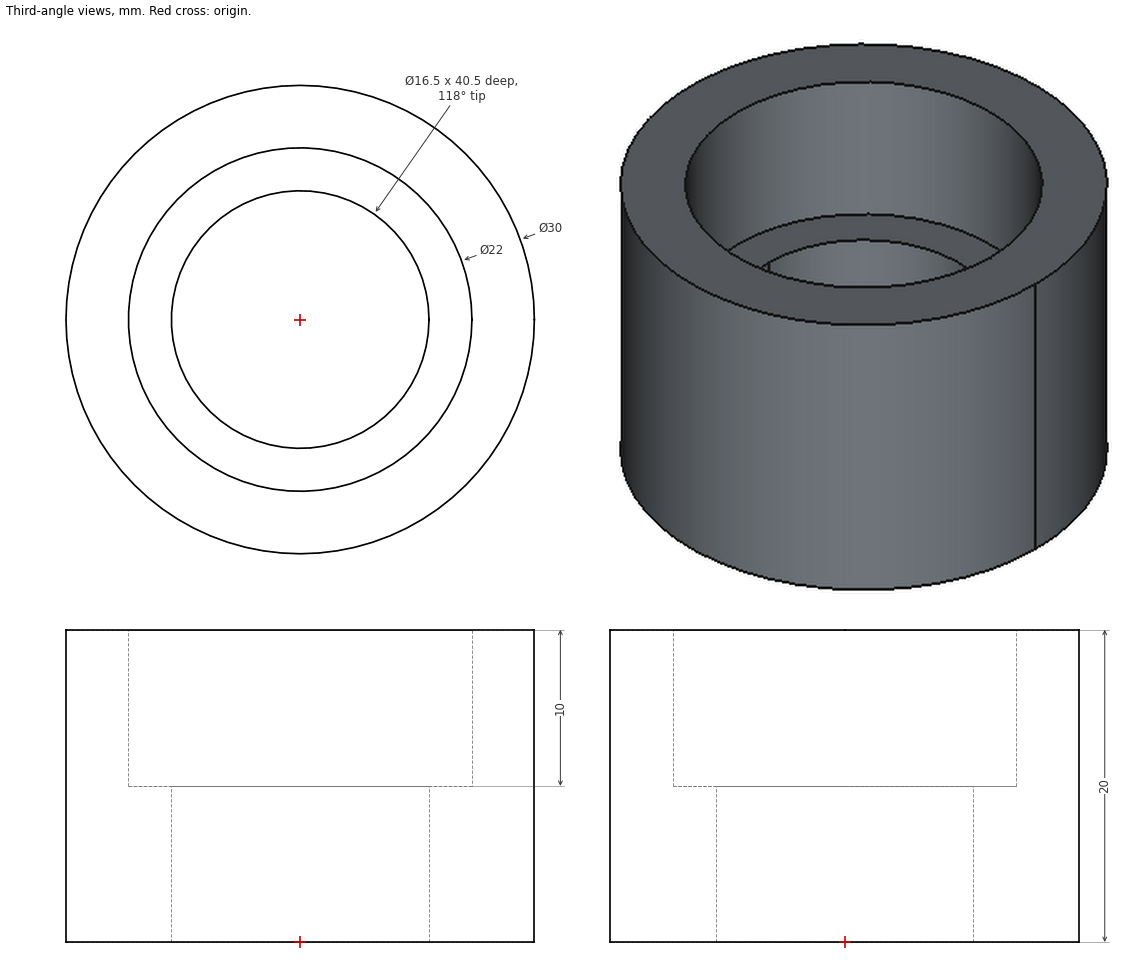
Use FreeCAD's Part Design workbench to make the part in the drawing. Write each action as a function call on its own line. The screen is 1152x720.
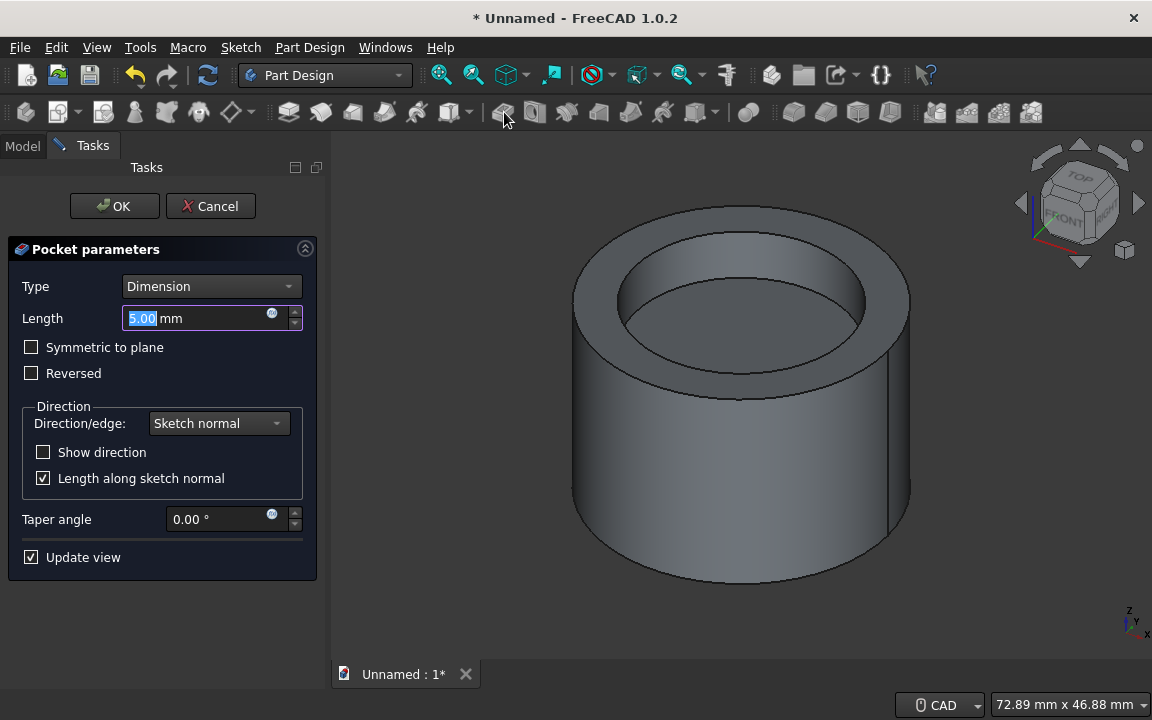
text(10)
key(Tab)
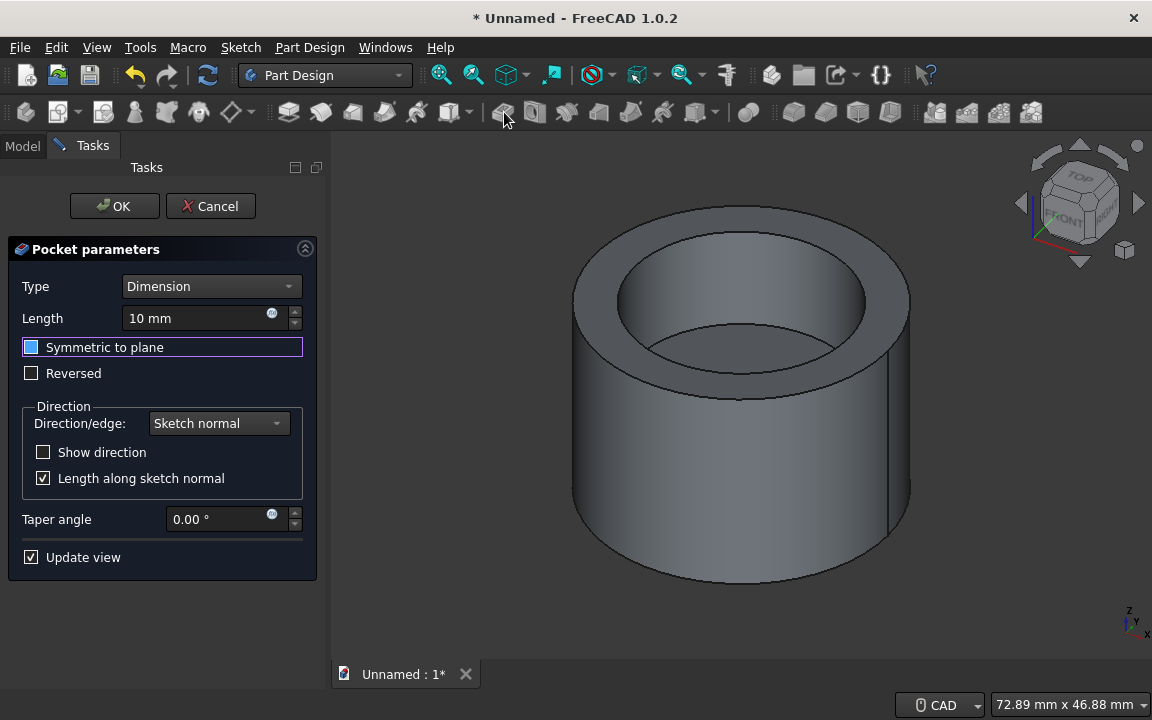
click(115, 206)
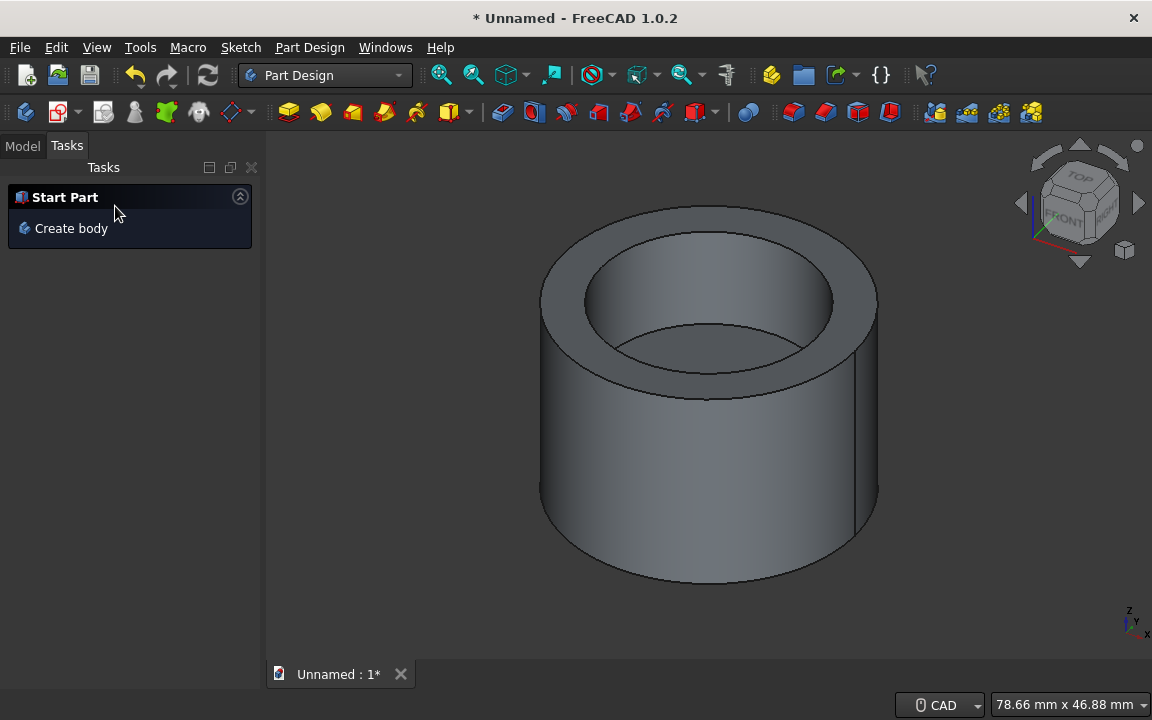
key(5)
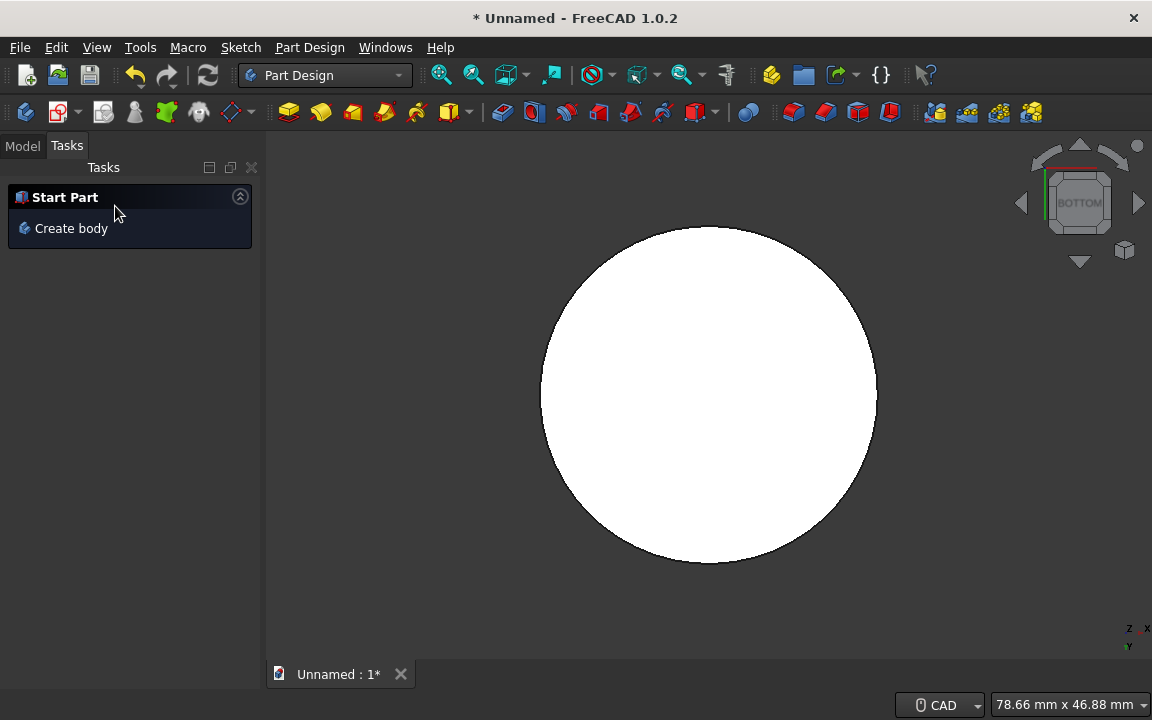
click(709, 394)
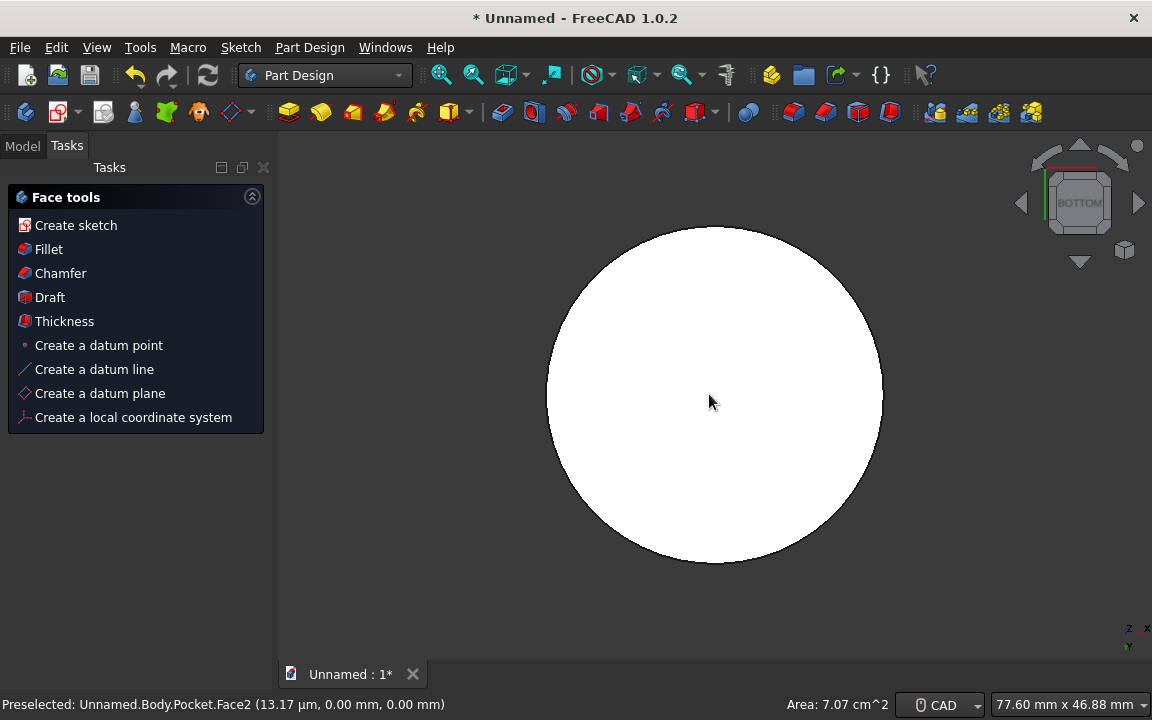
click(58, 112)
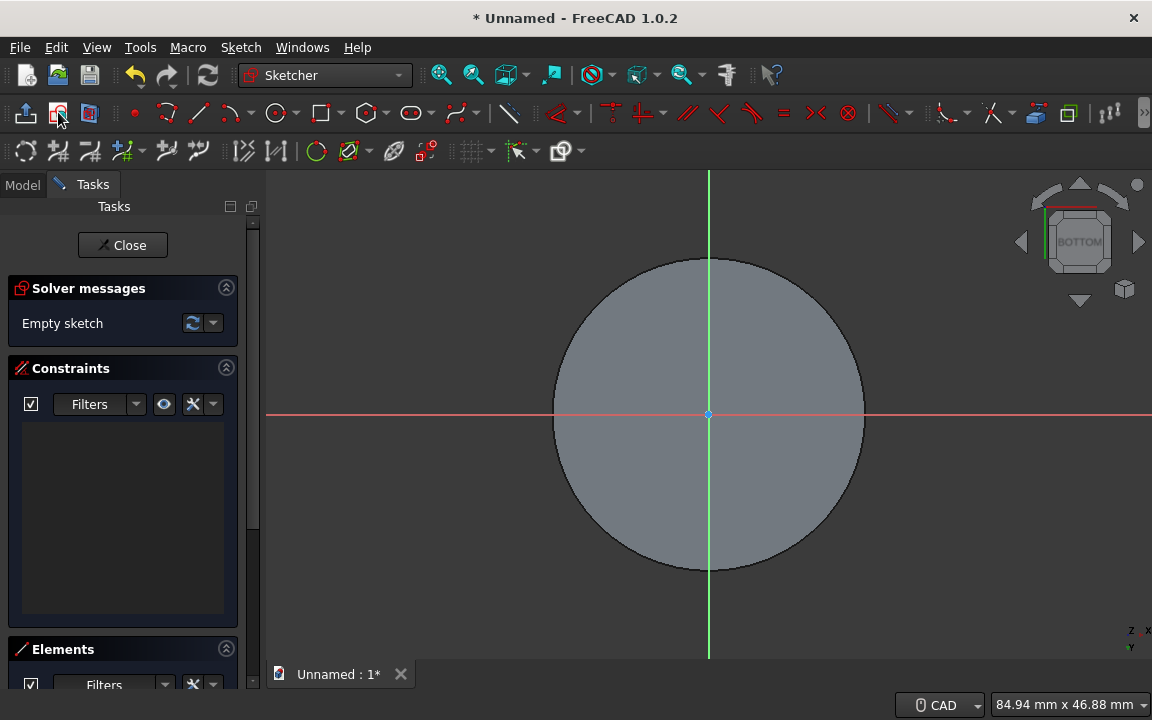
scroll(792, 415, up, 3)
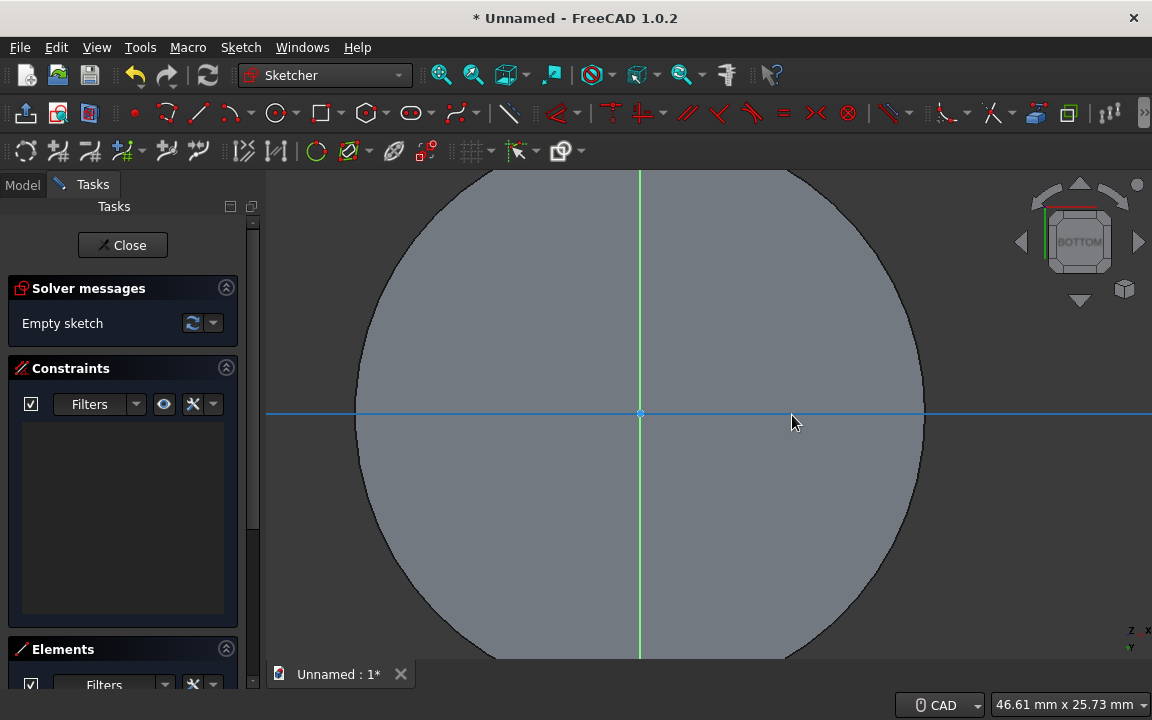
click(276, 114)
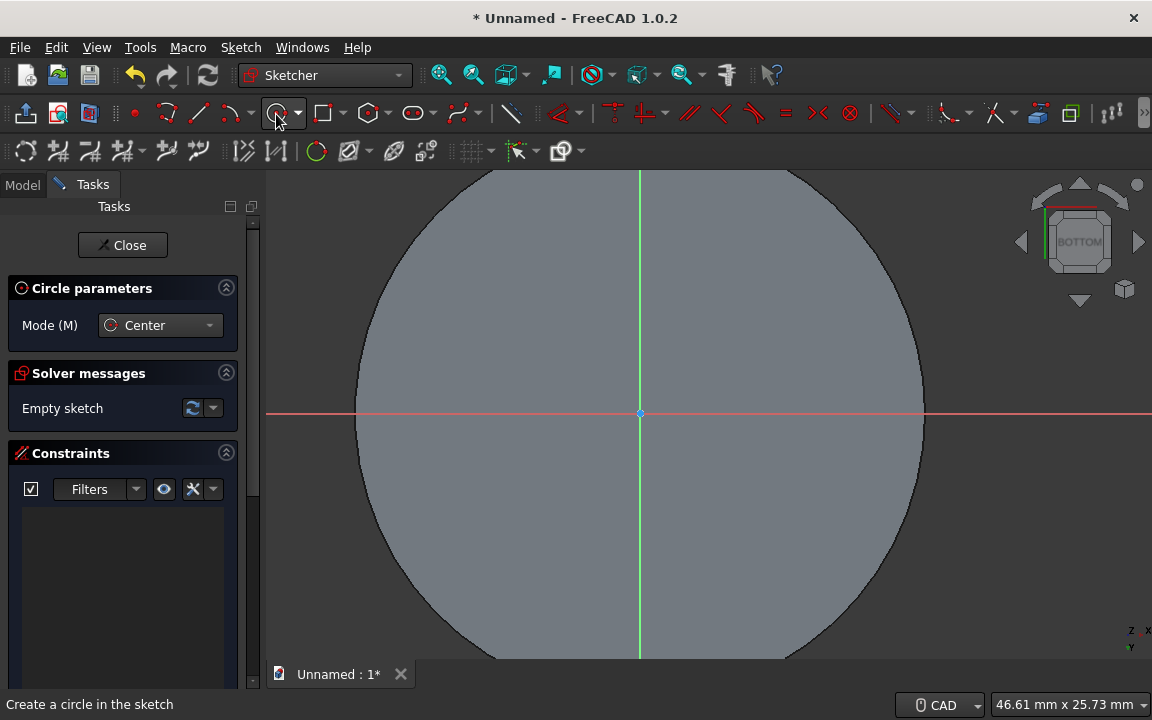
click(640, 414)
click(751, 303)
key(Escape)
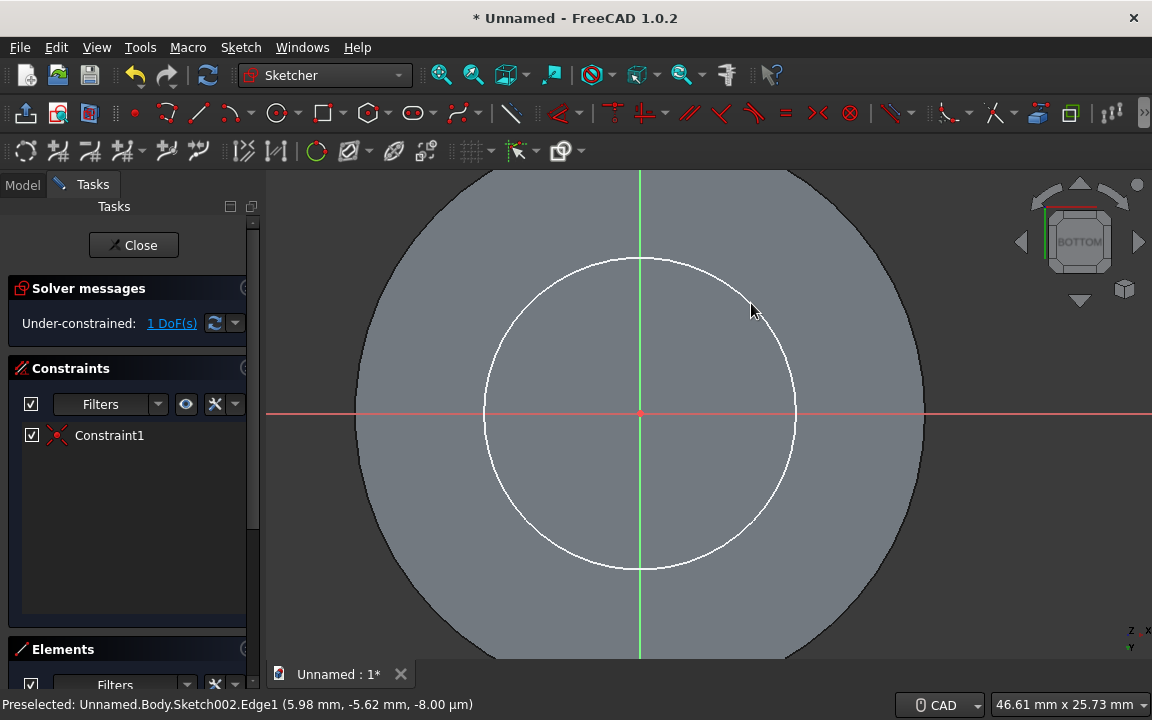
click(558, 114)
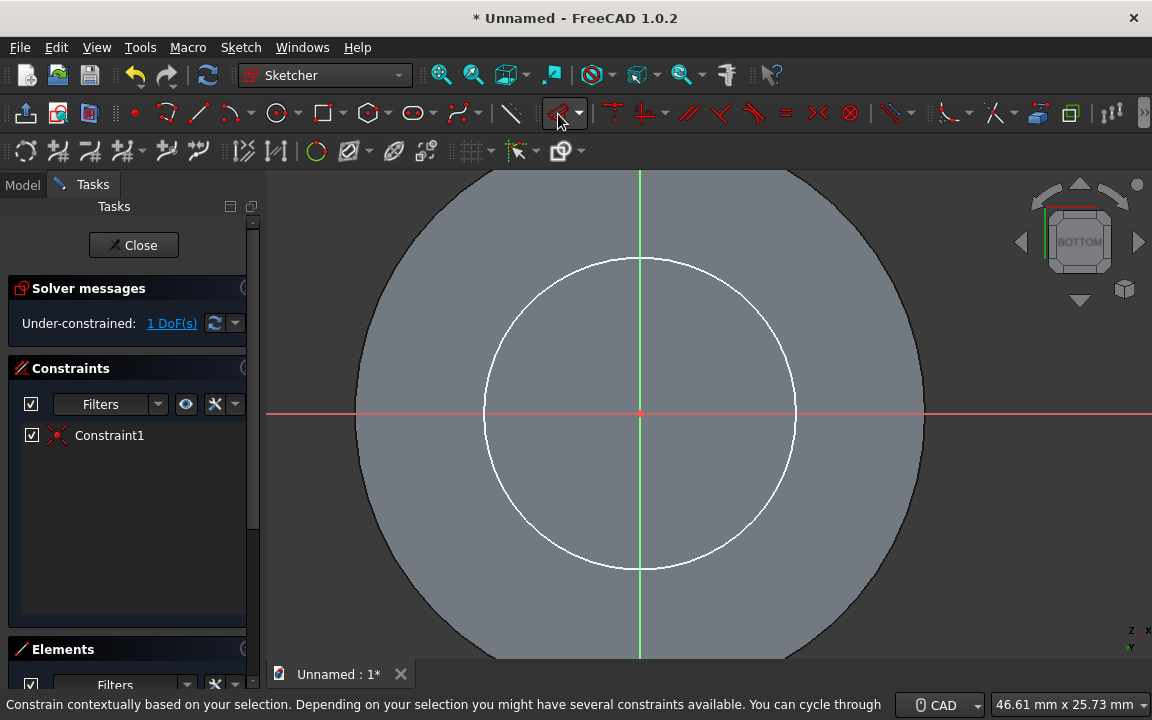
click(750, 303)
click(773, 280)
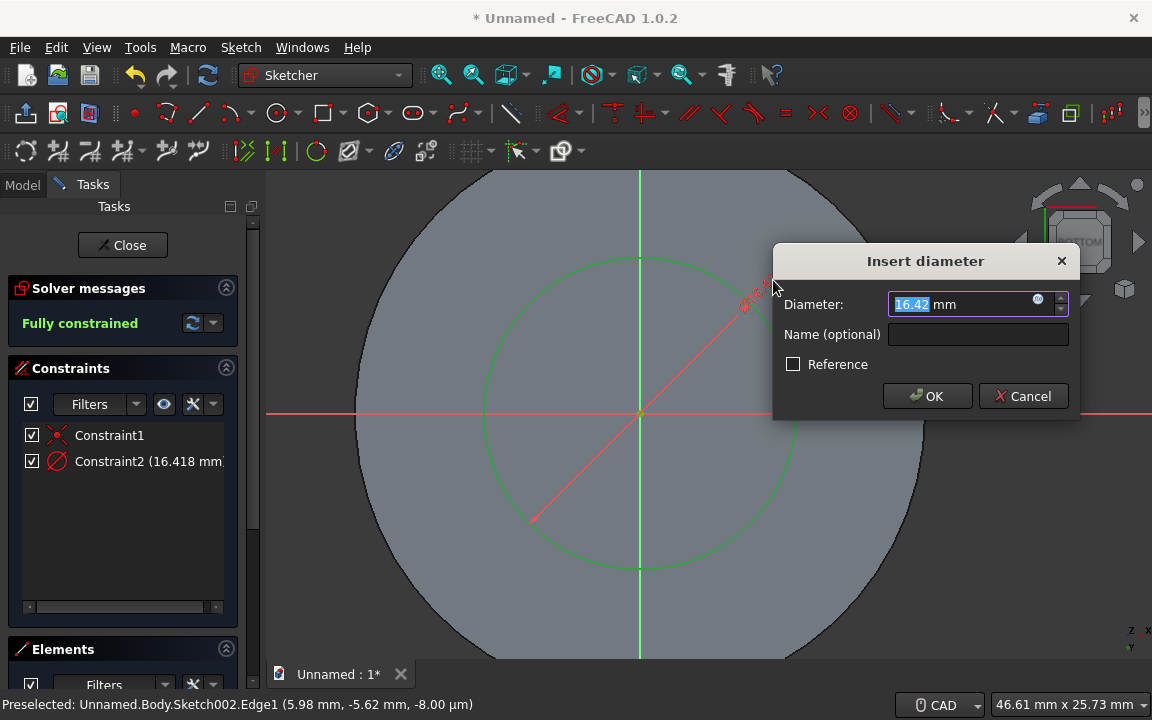
text(16.5)
key(Return)
key(Escape)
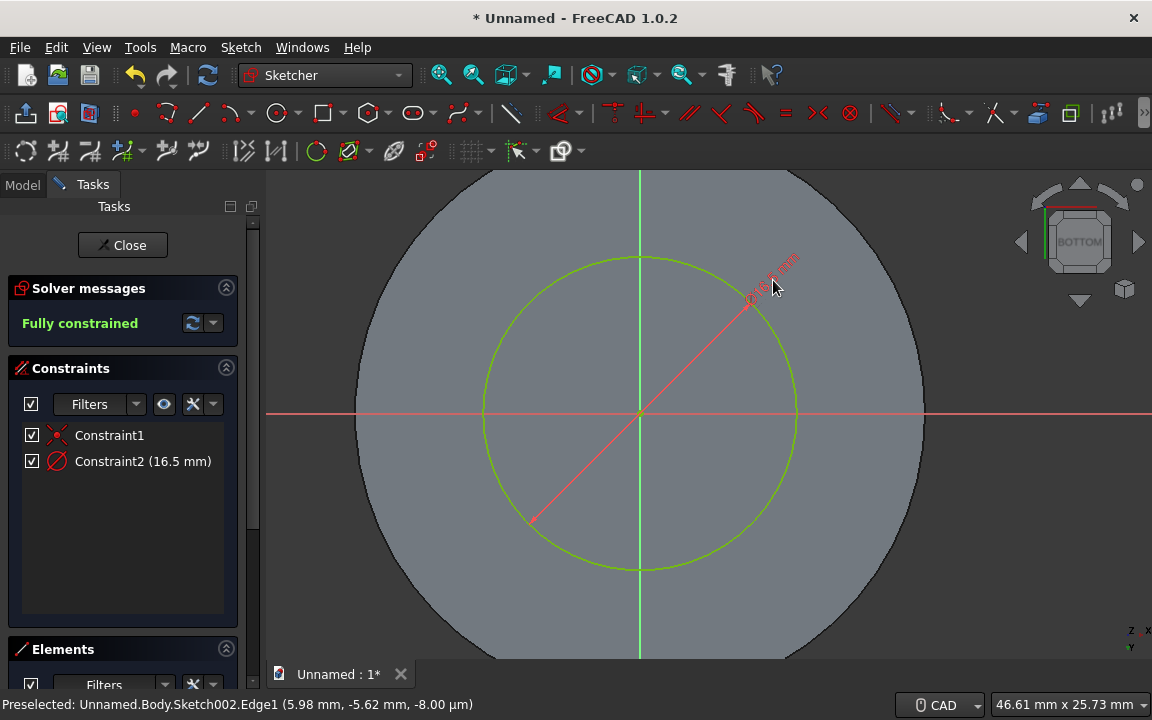
click(123, 245)